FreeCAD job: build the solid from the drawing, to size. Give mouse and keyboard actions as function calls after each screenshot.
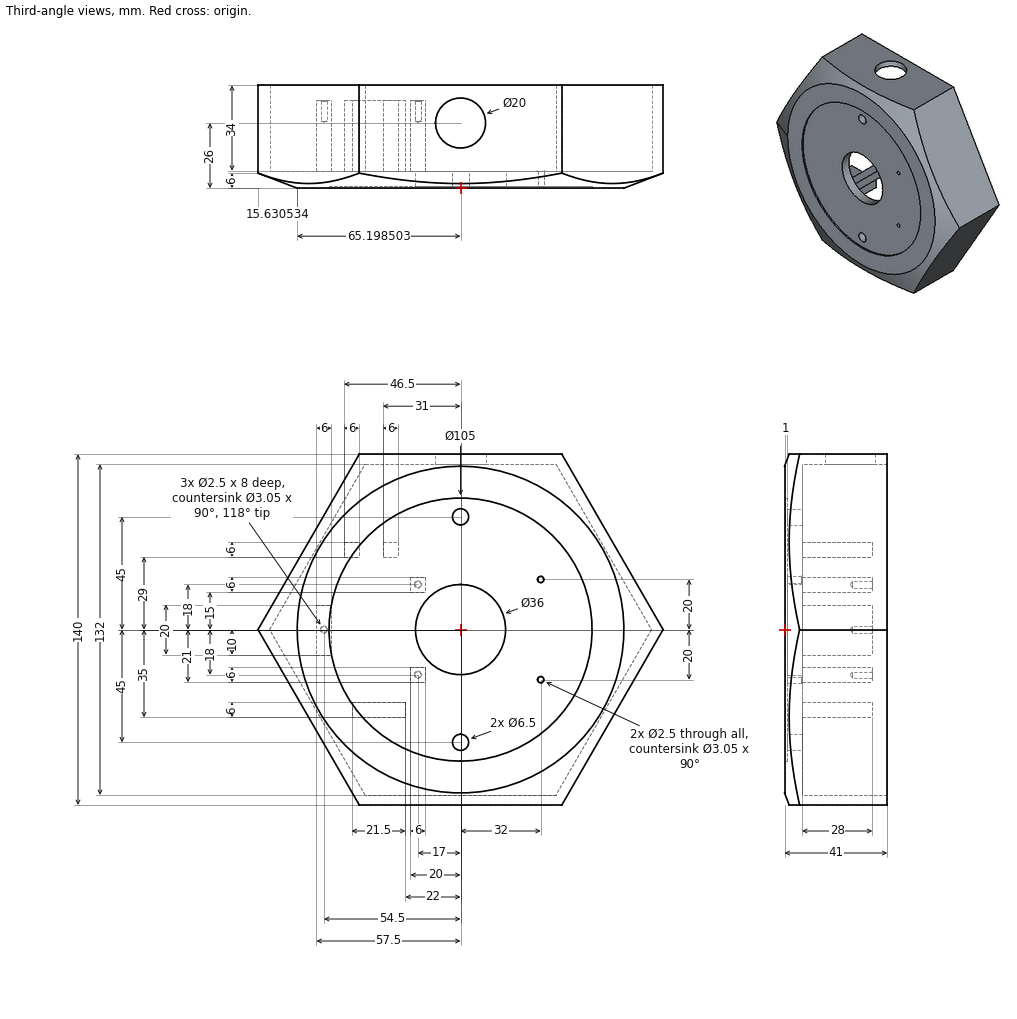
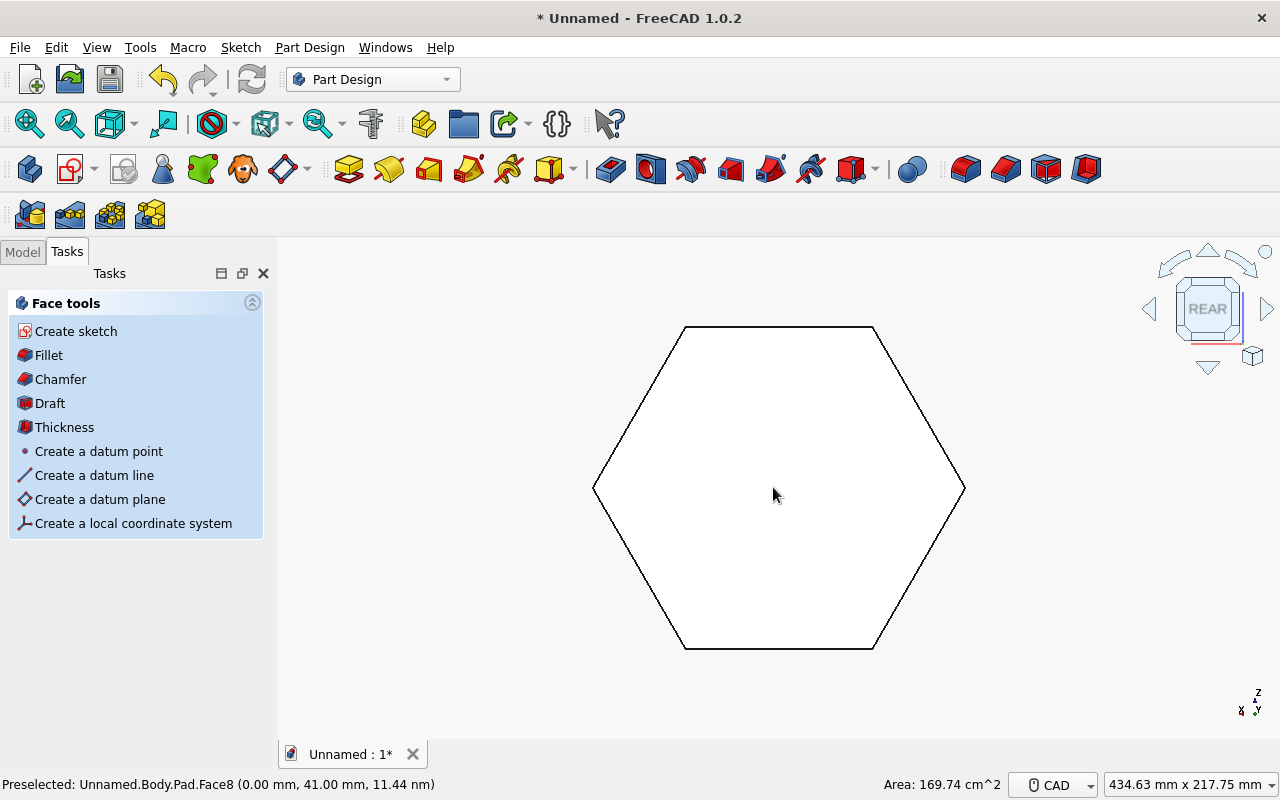
click(70, 170)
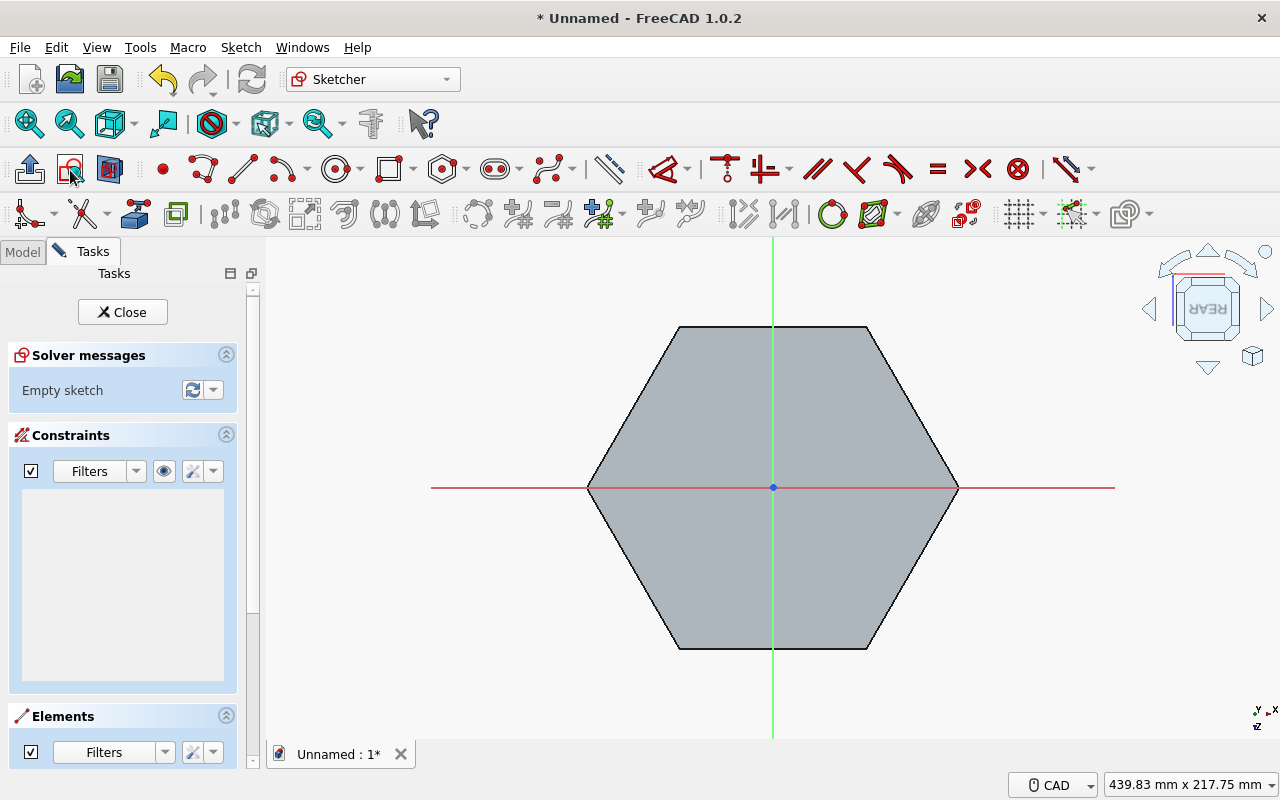
key(g)
key(p)
key(6)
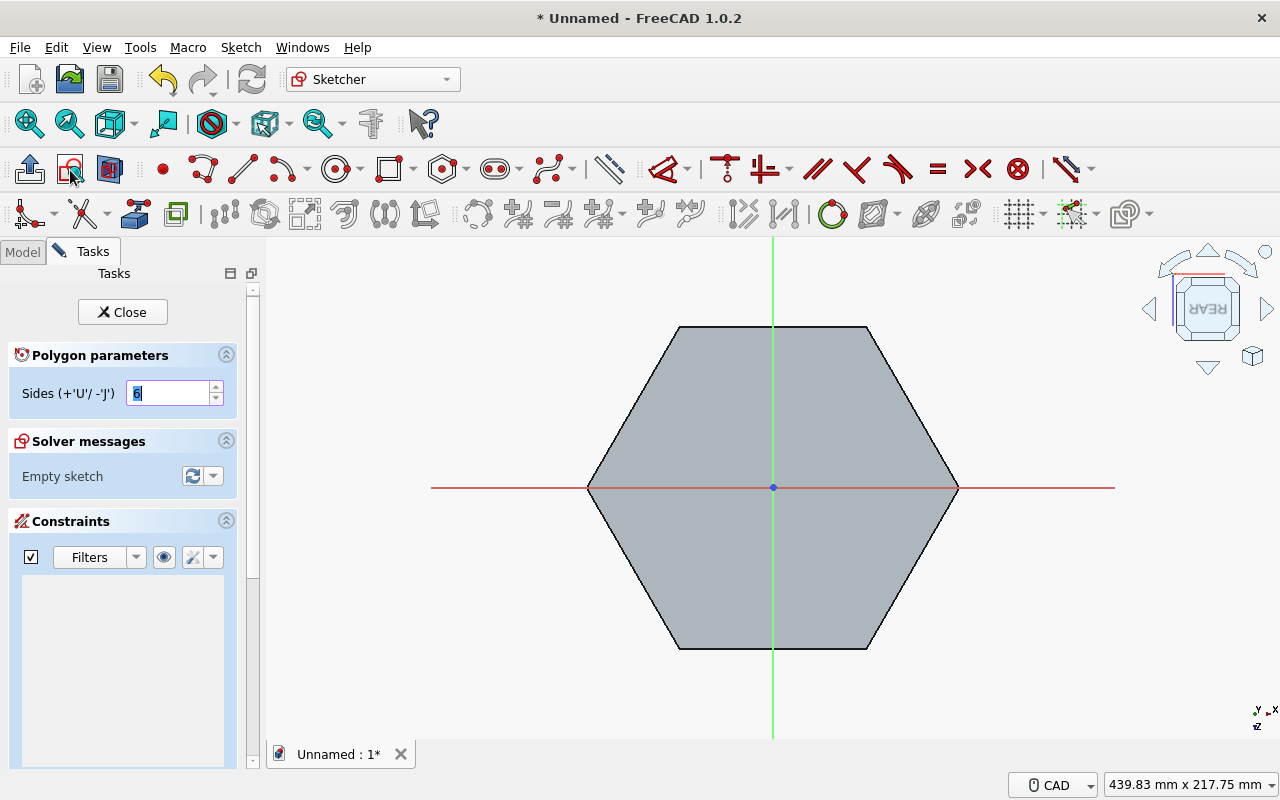
click(773, 488)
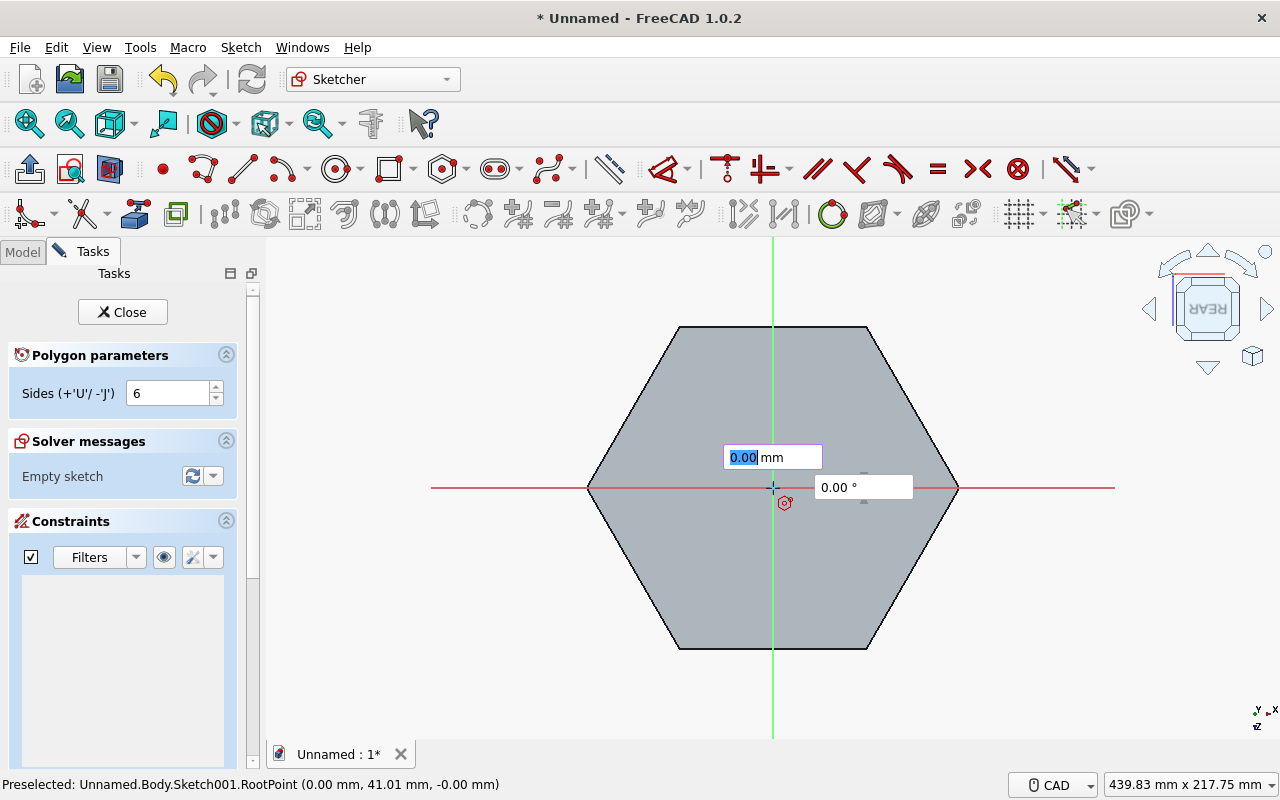
click(949, 488)
right_click(949, 488)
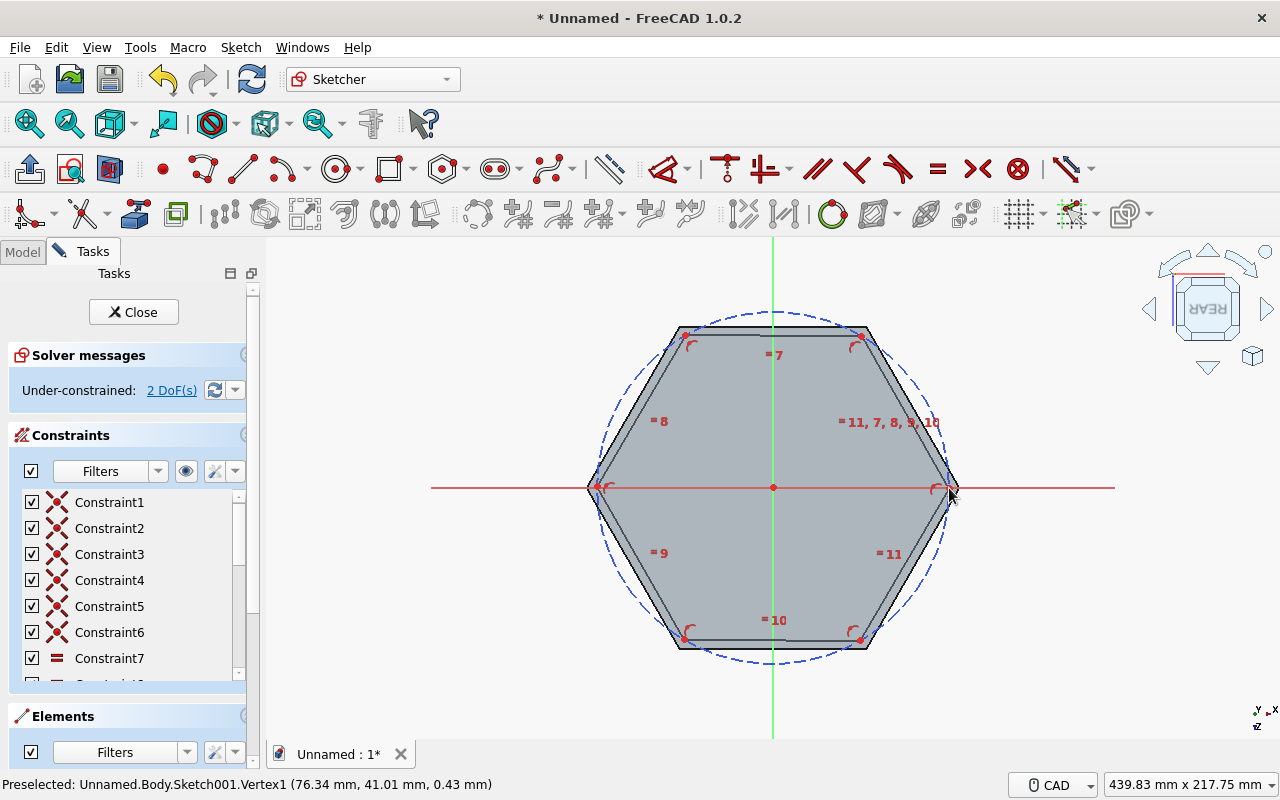
click(809, 336)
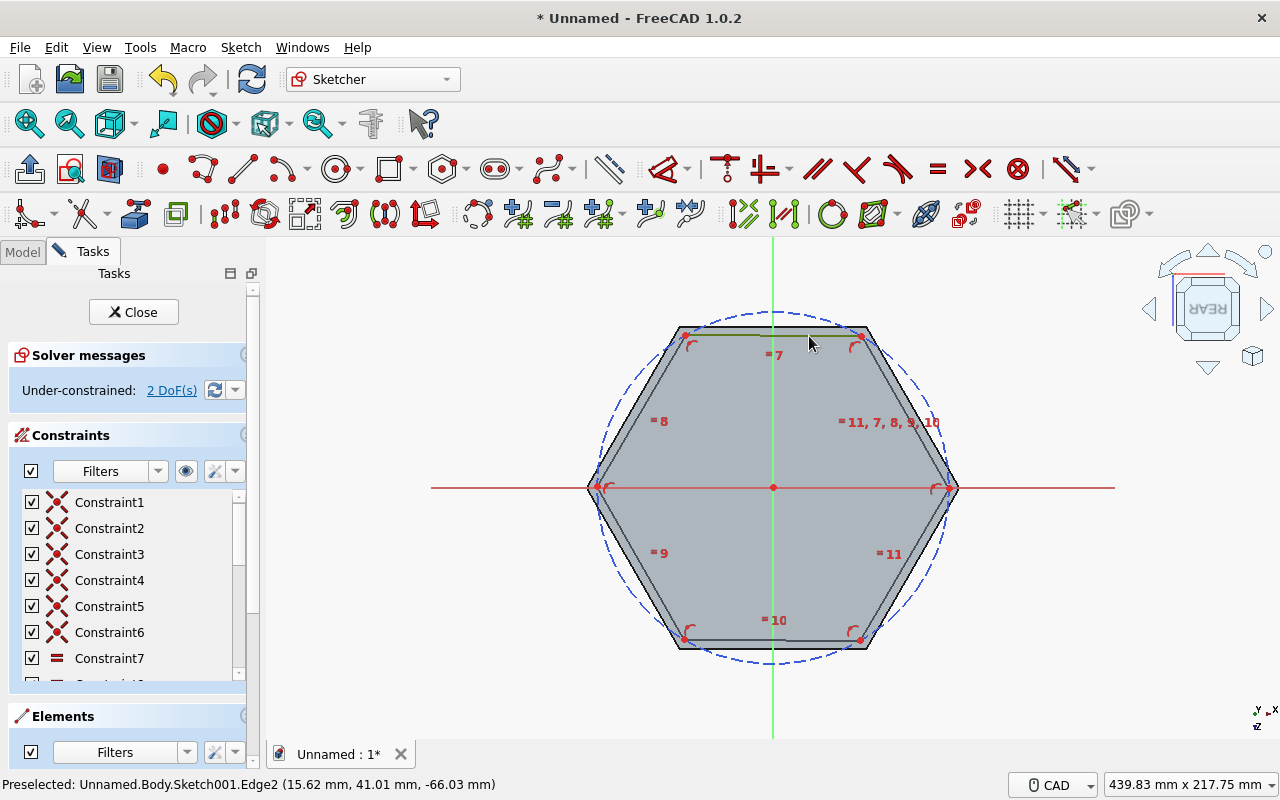
key(h)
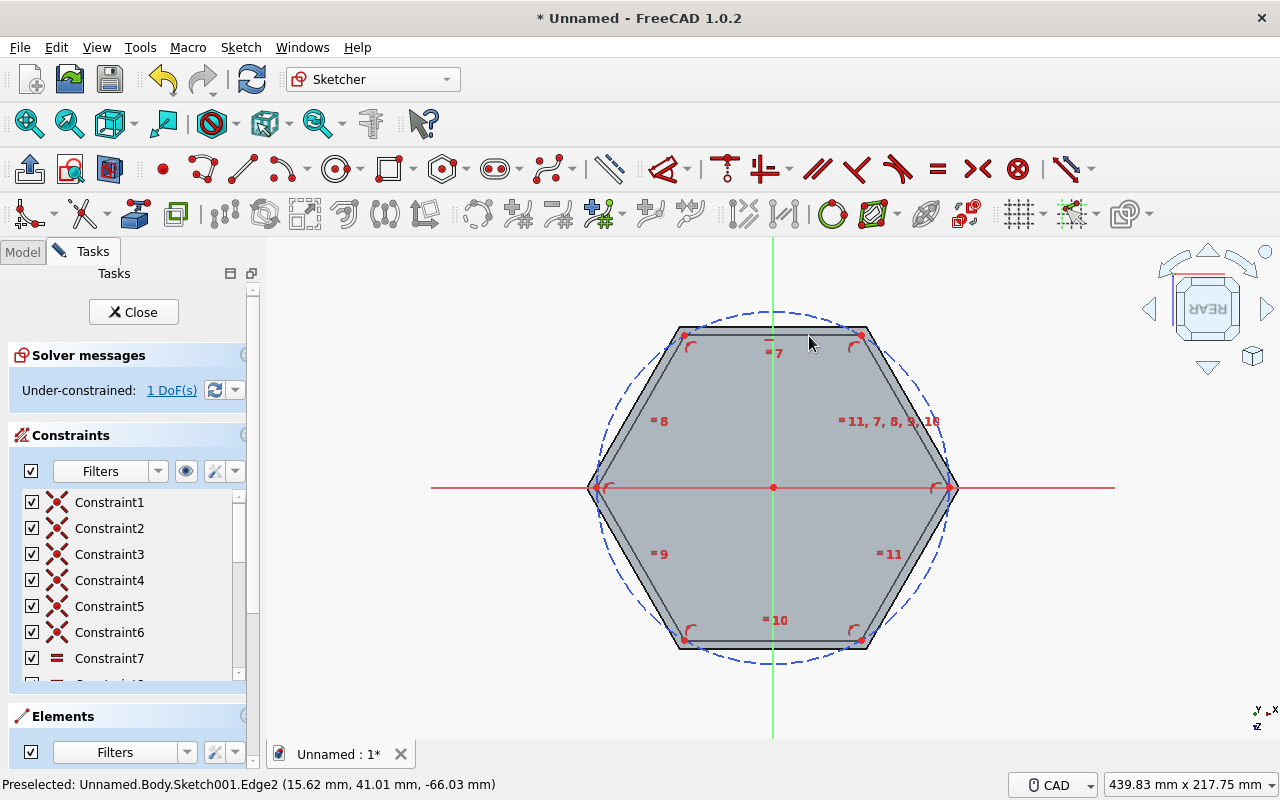
click(685, 641)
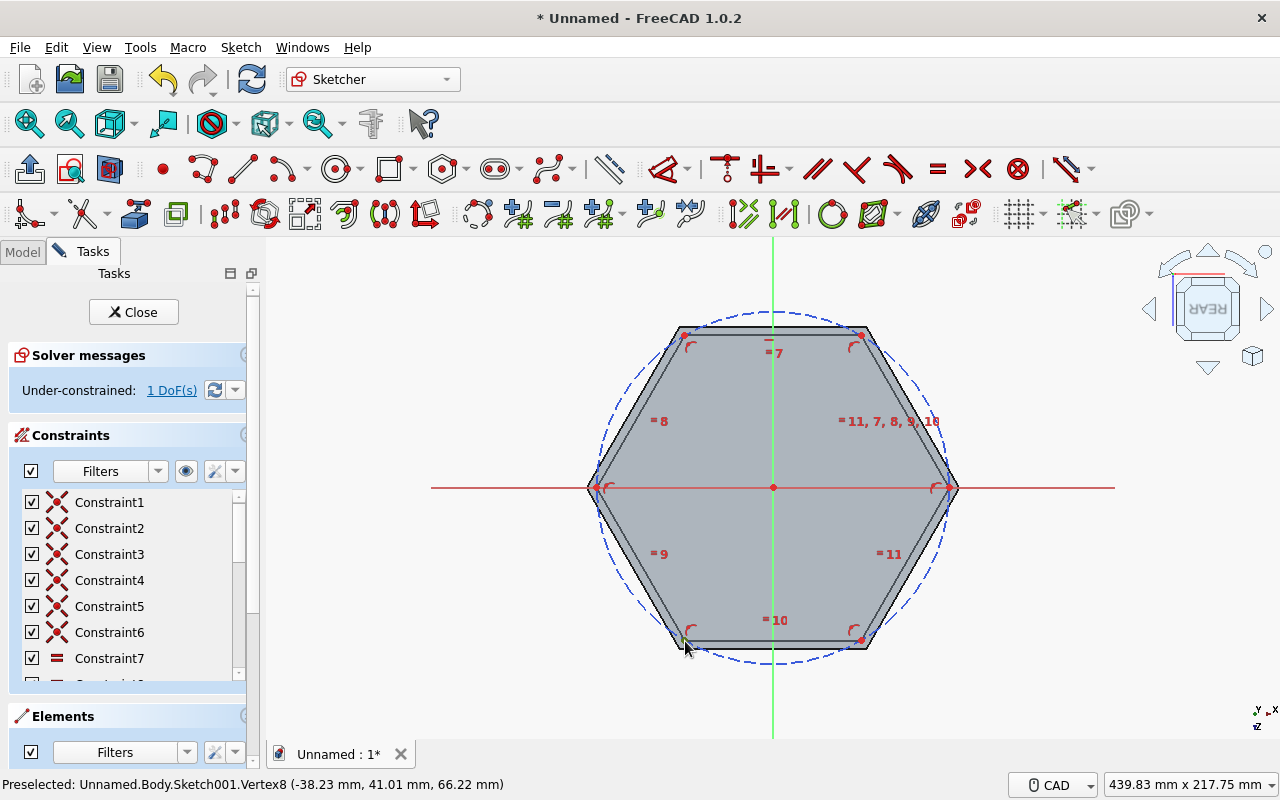
click(861, 335)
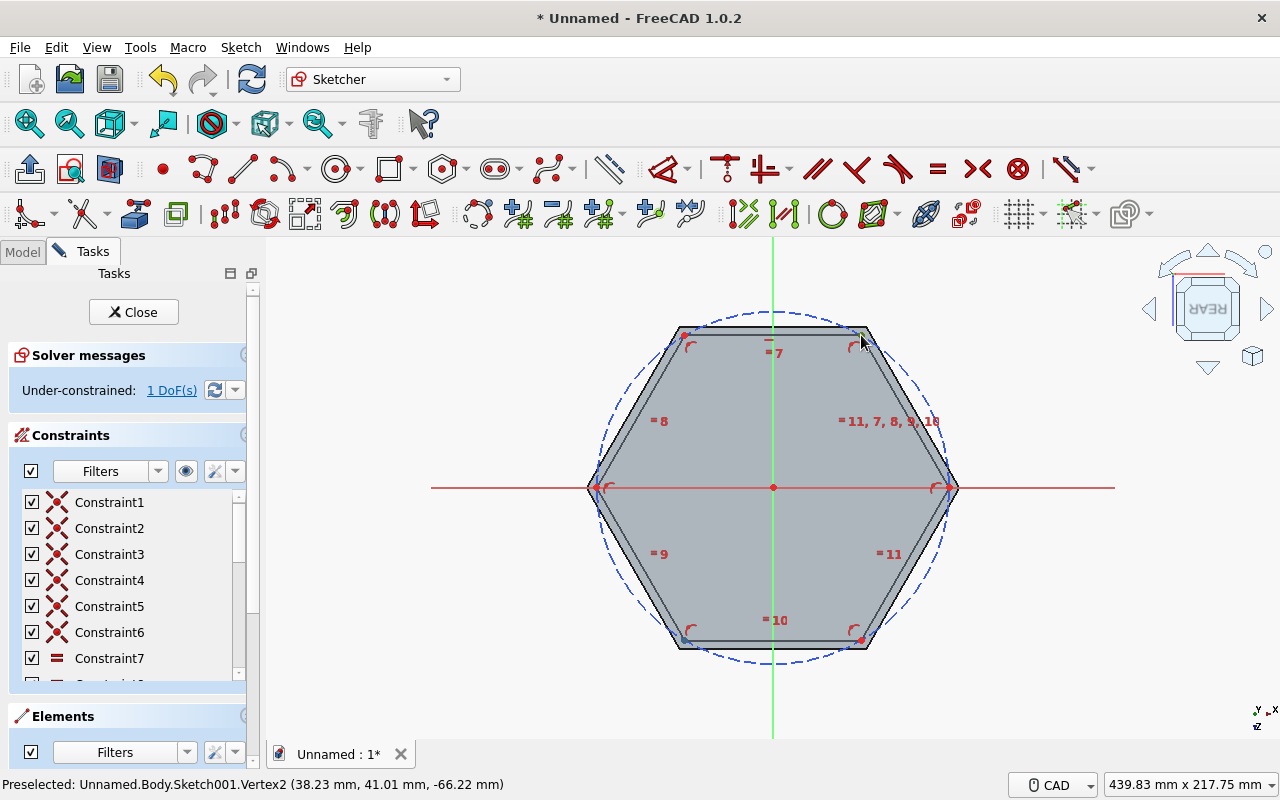
key(i)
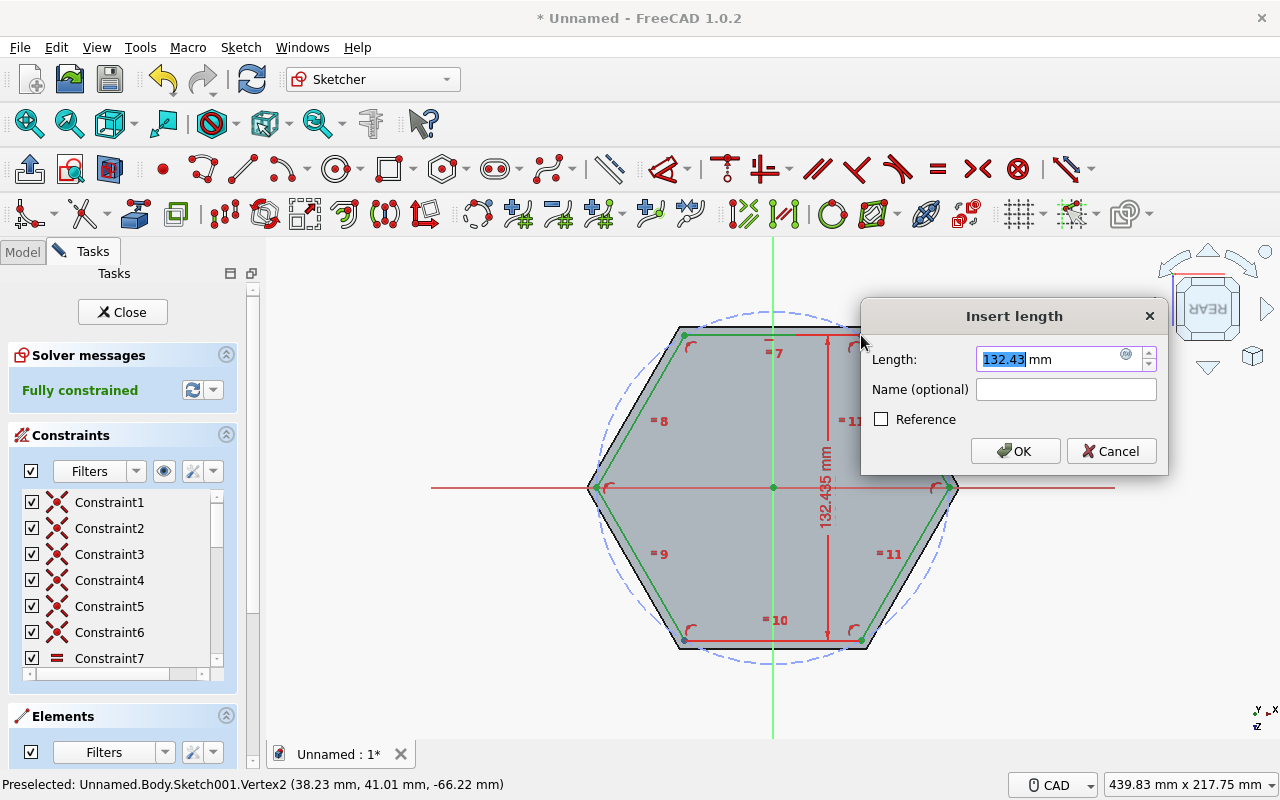
text(132)
key(Return)